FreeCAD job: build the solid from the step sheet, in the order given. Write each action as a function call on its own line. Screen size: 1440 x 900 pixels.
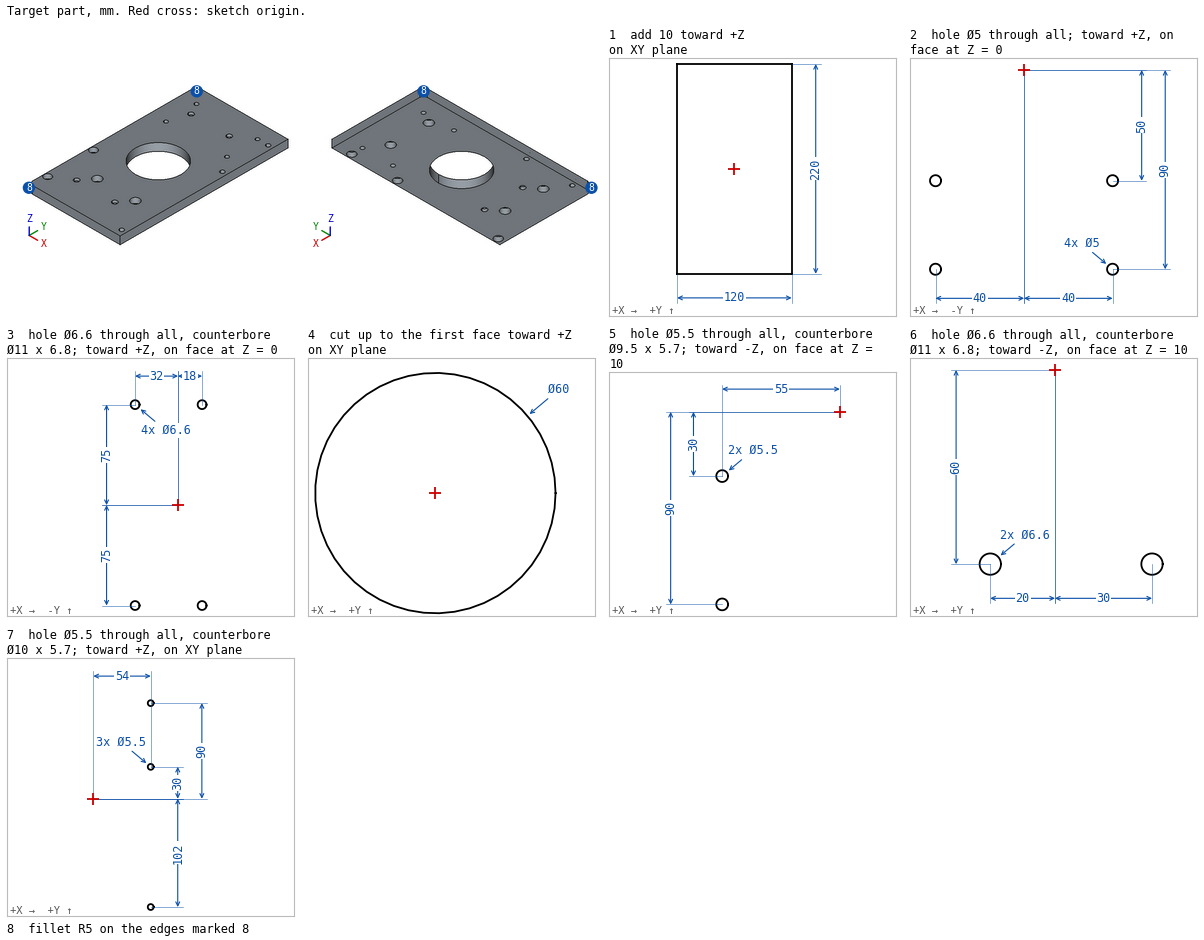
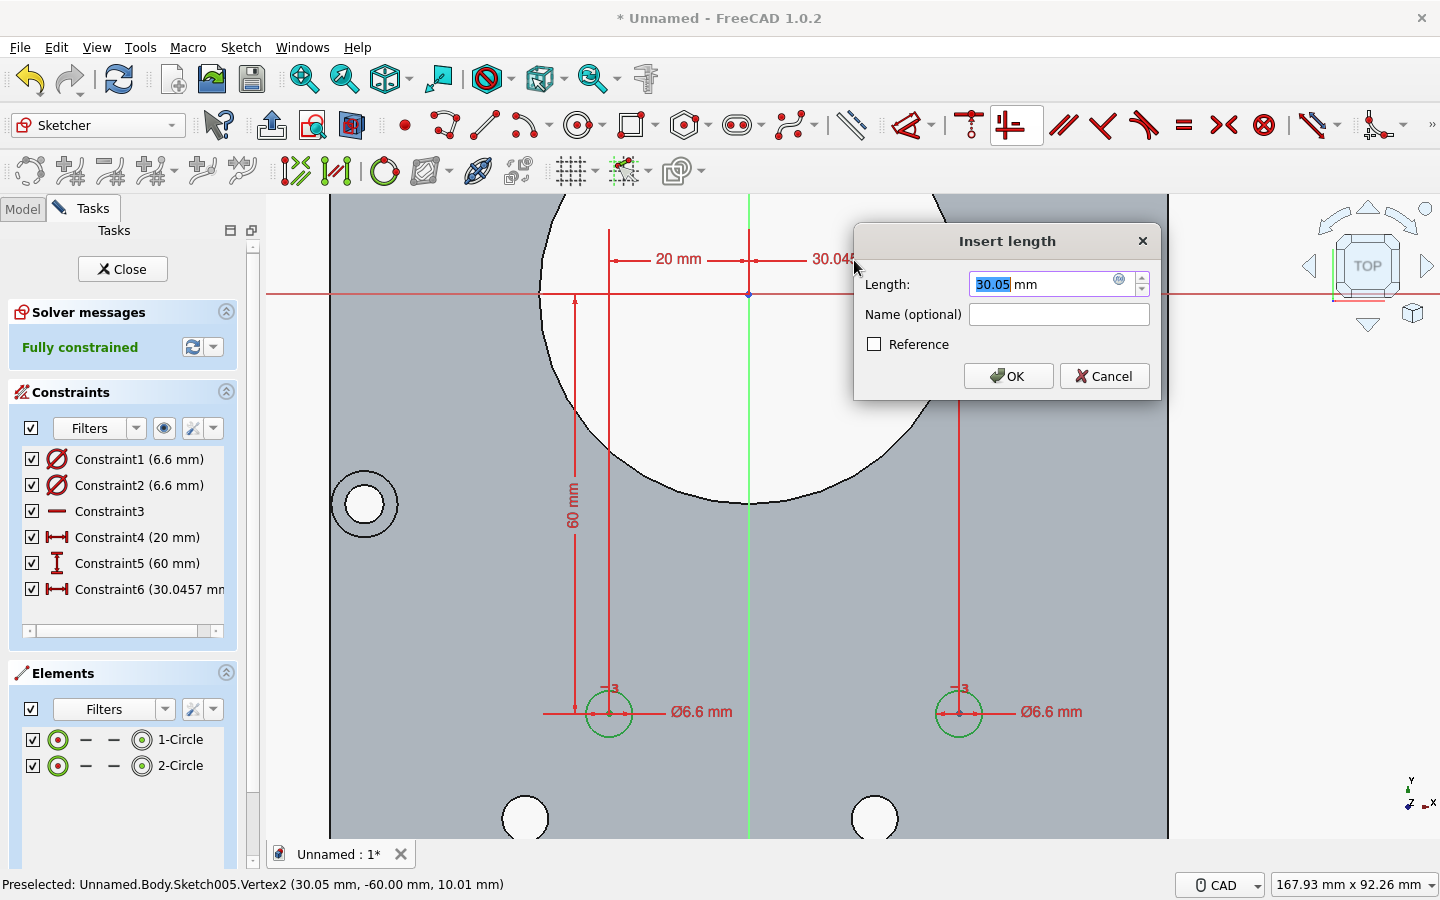
text(30)
key(Return)
key(Escape)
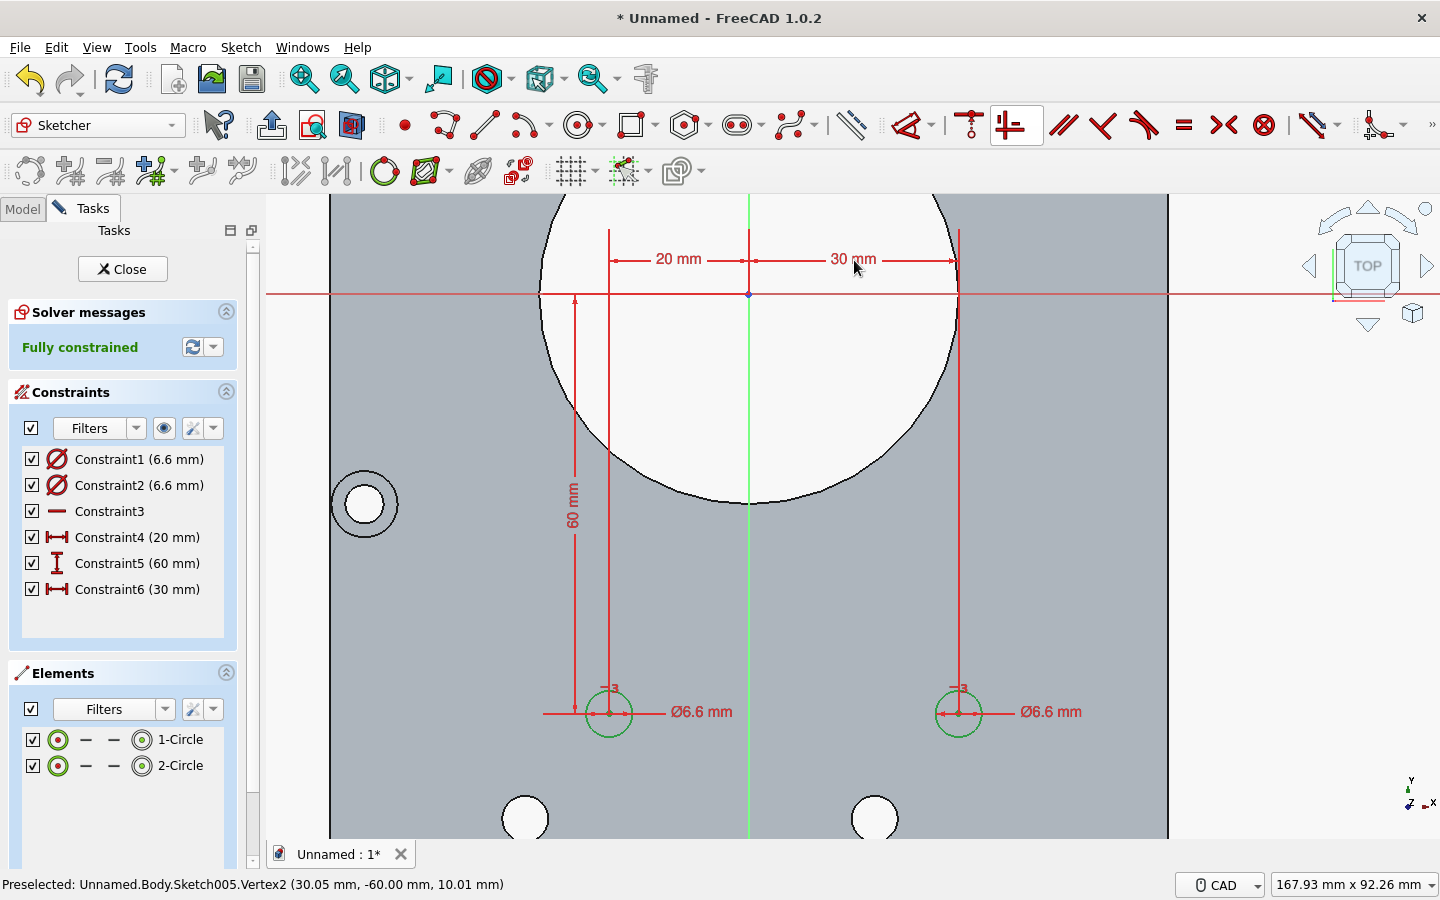
click(123, 269)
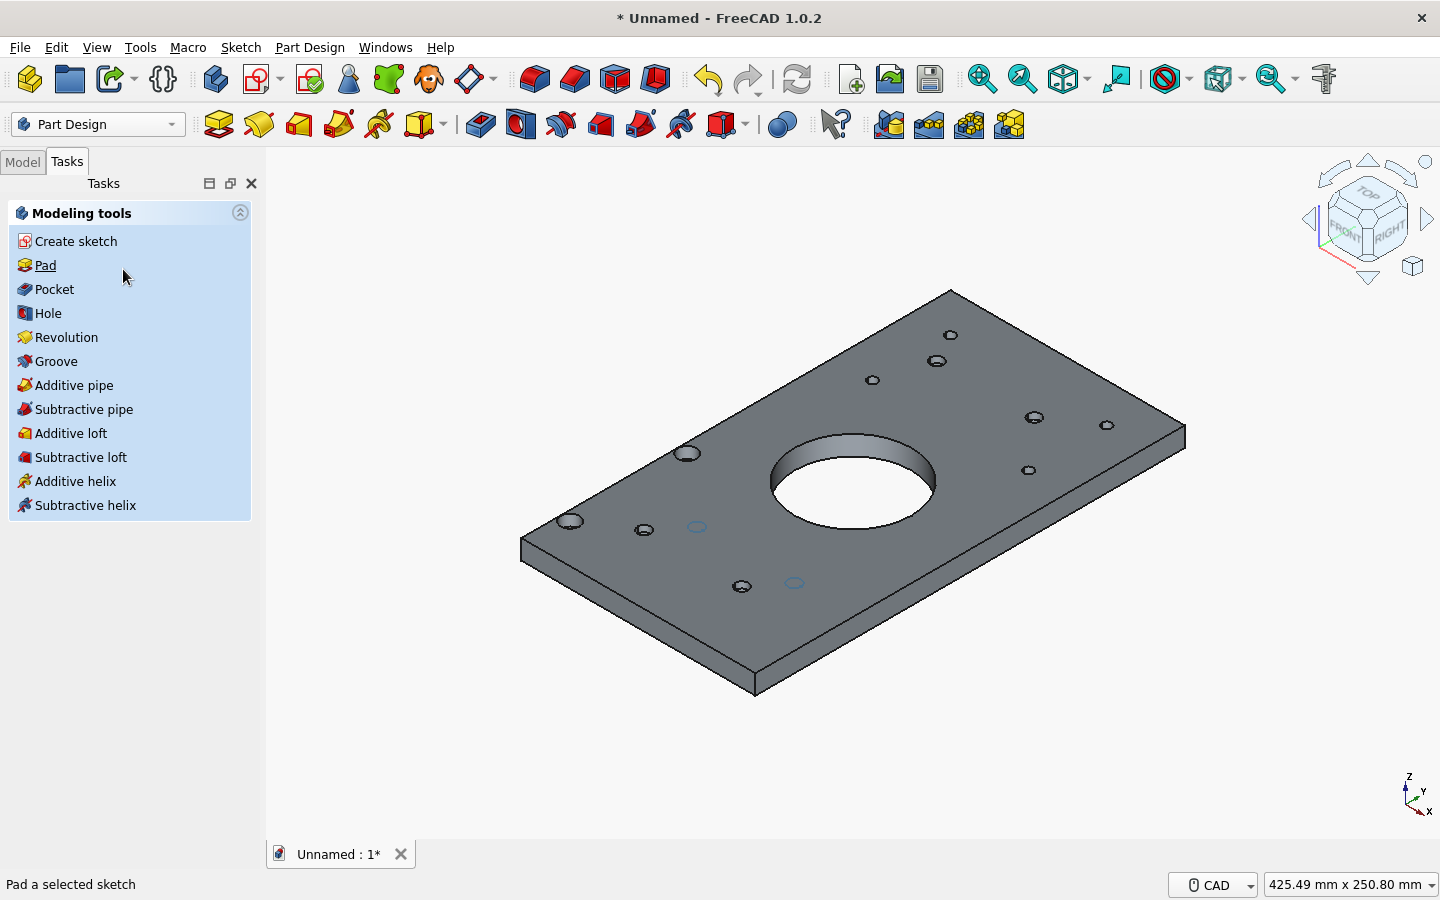
click(522, 124)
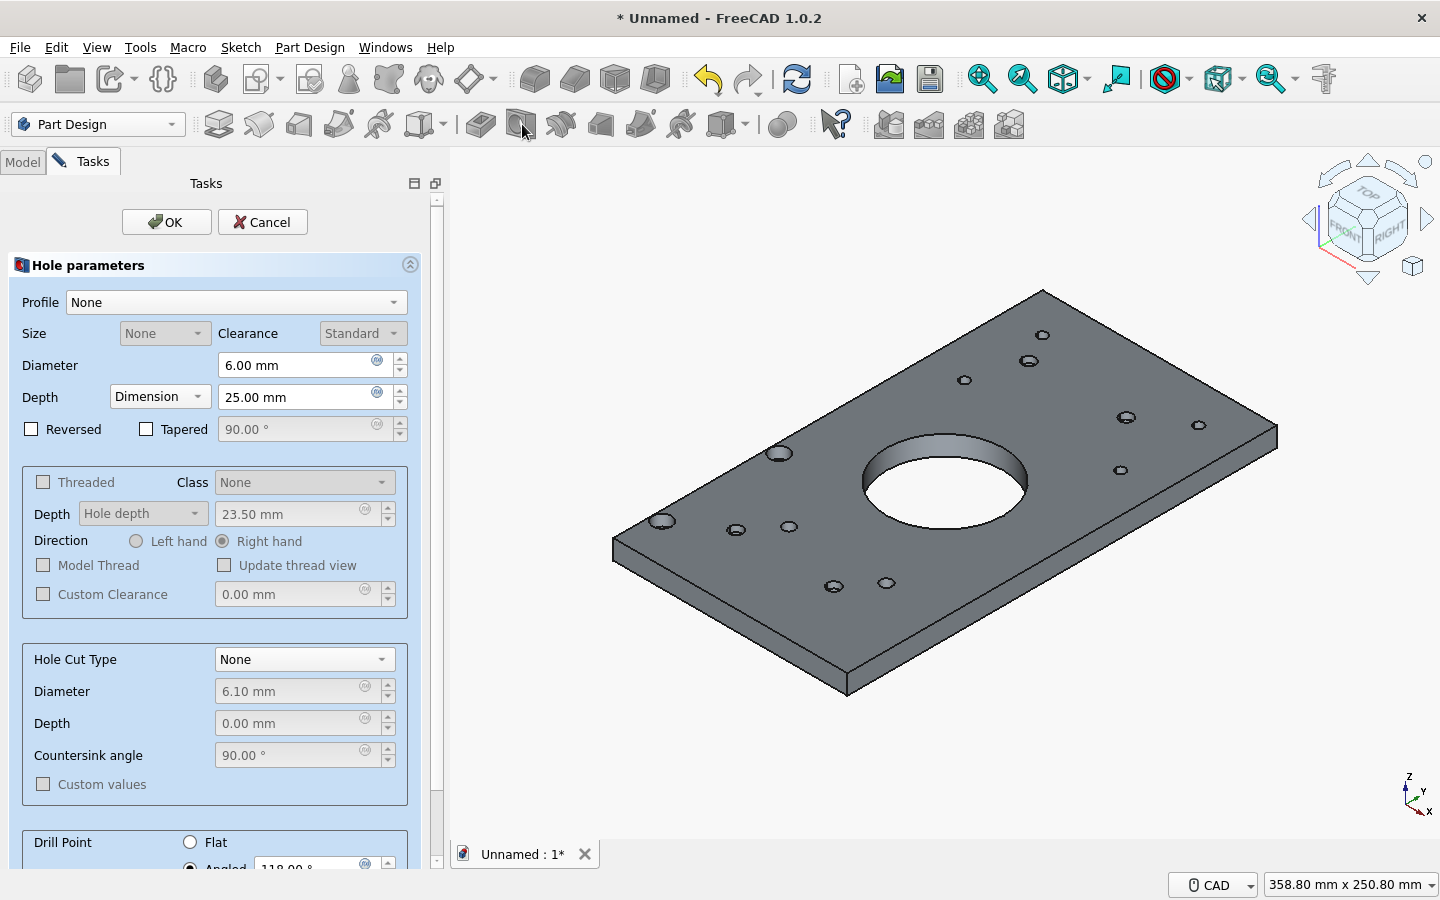
triple_click(305, 365)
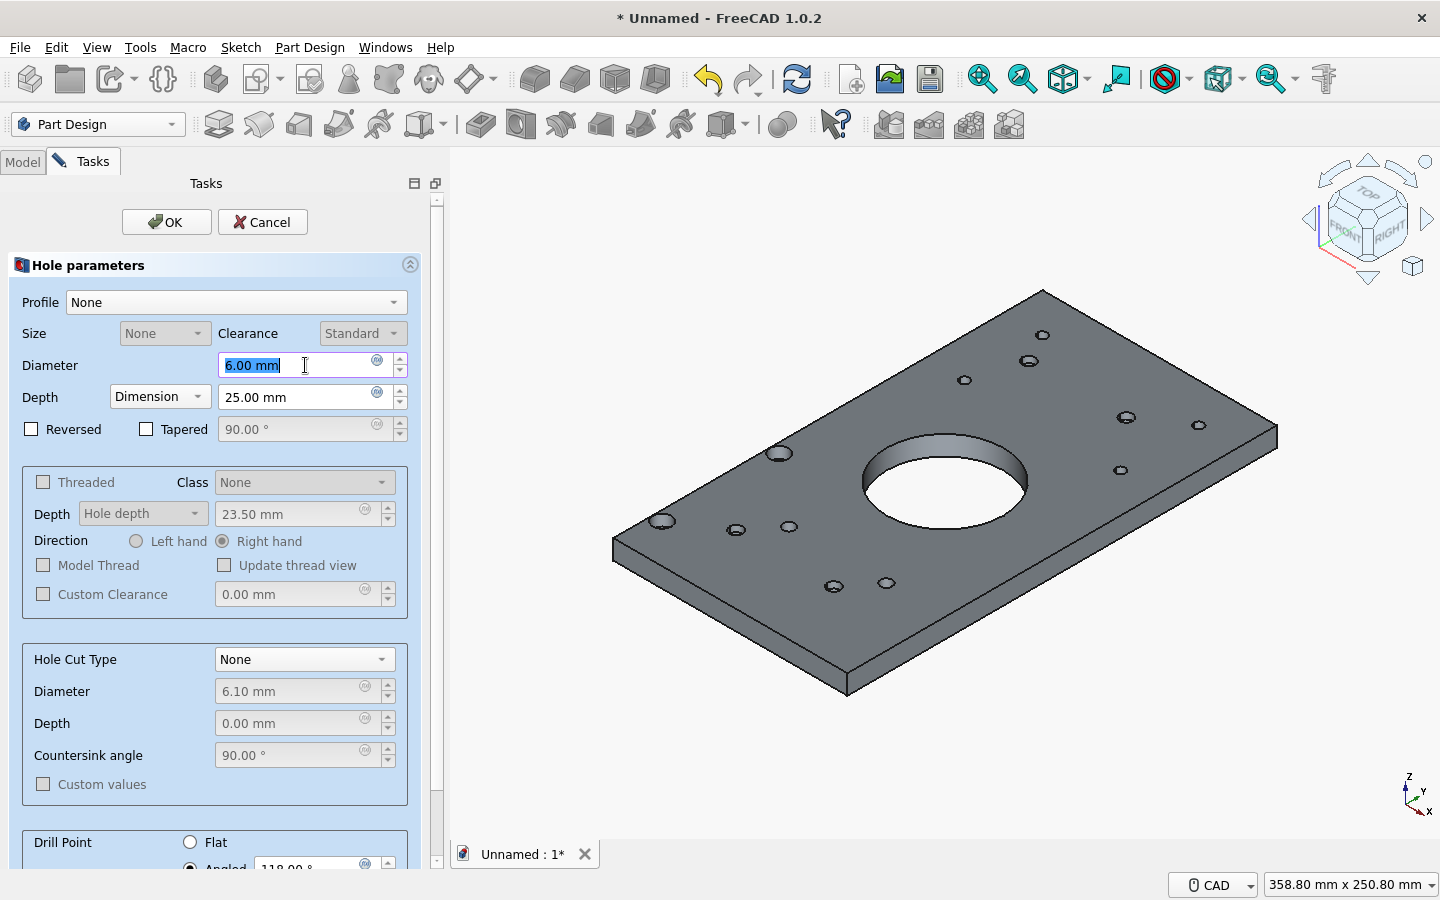
text(6.6)
key(Tab)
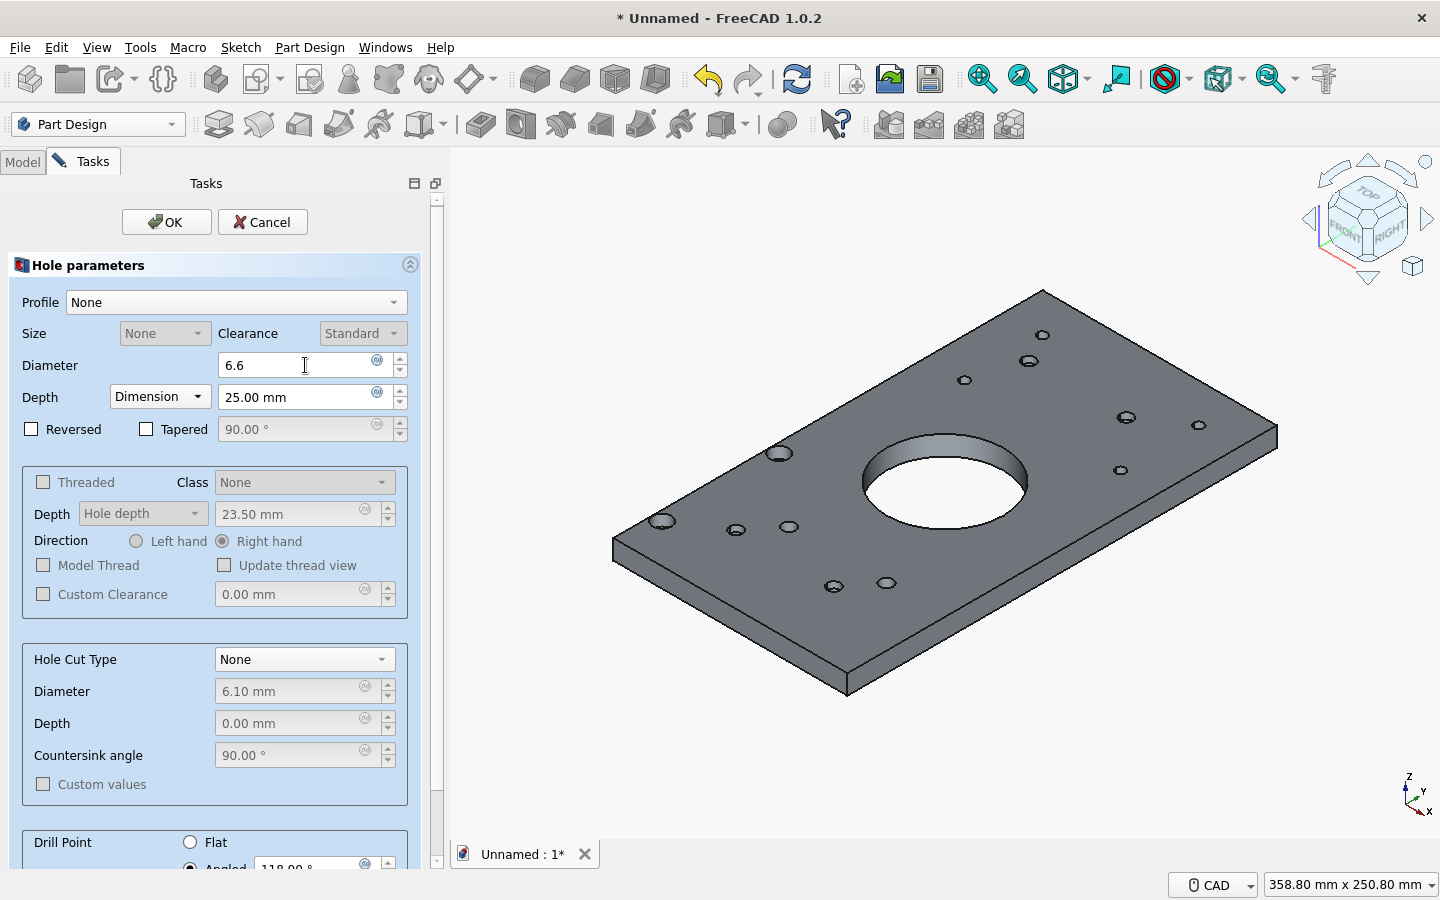
click(161, 396)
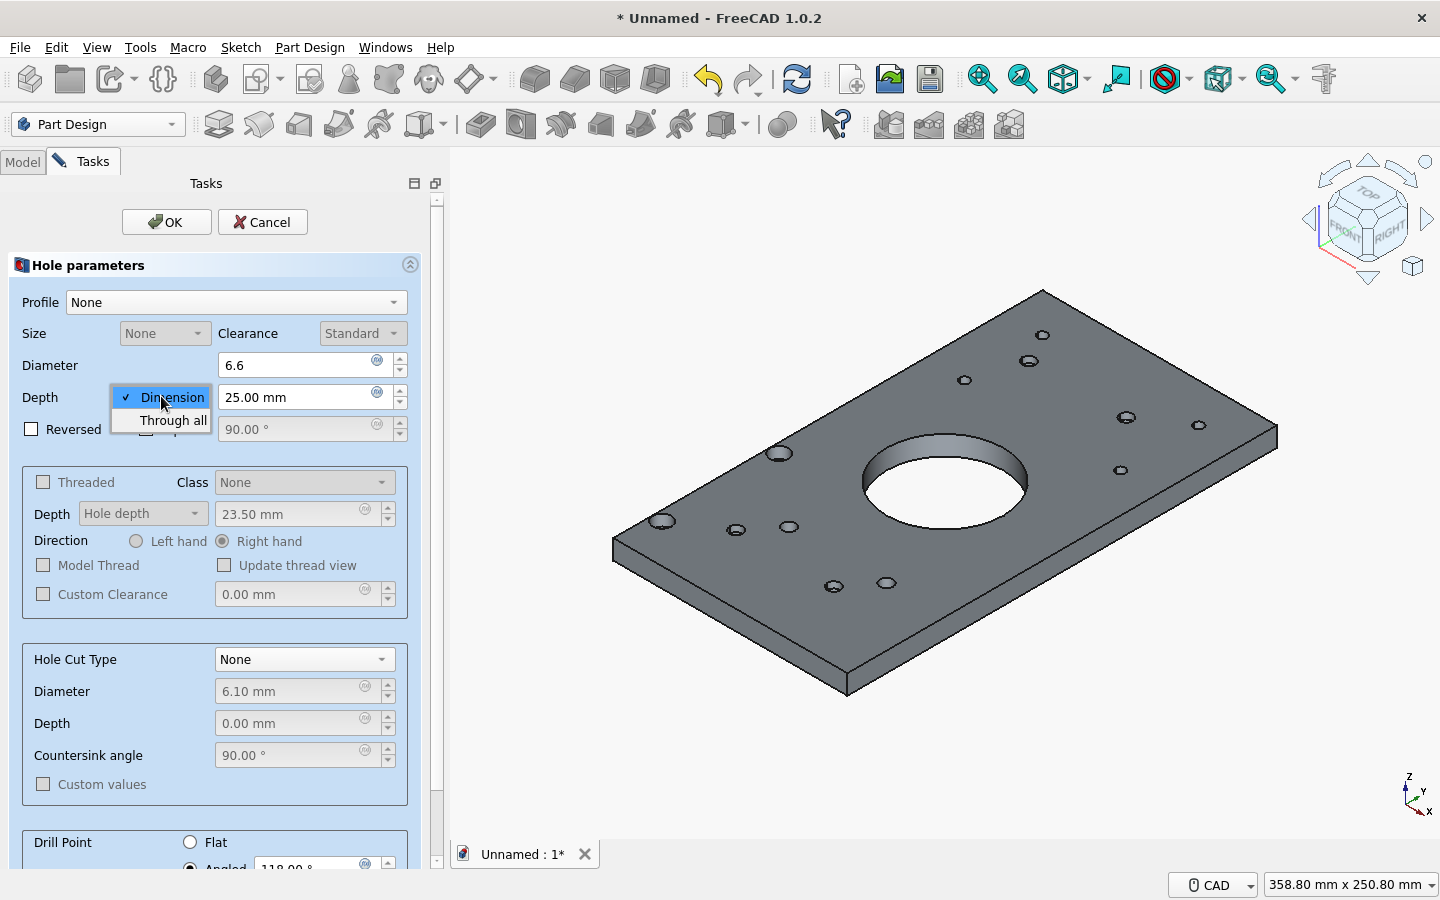
click(160, 420)